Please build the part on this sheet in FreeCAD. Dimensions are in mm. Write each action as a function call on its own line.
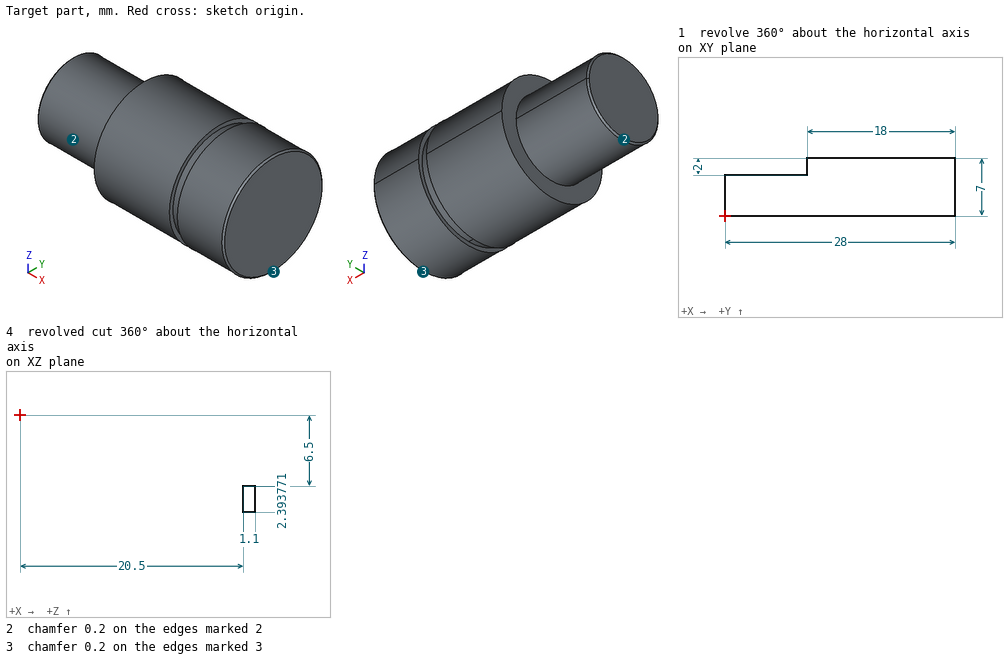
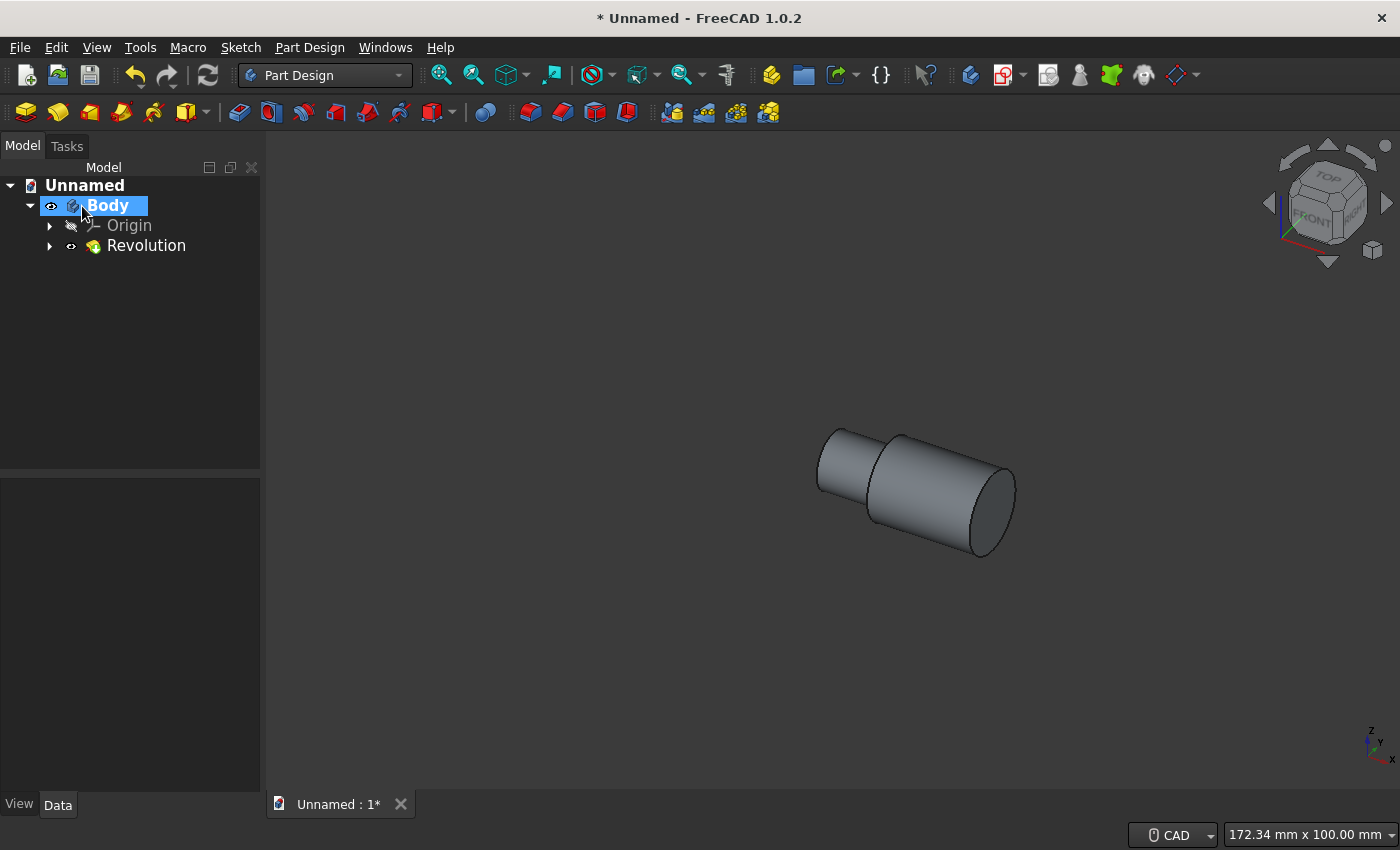
key(v)
key(f)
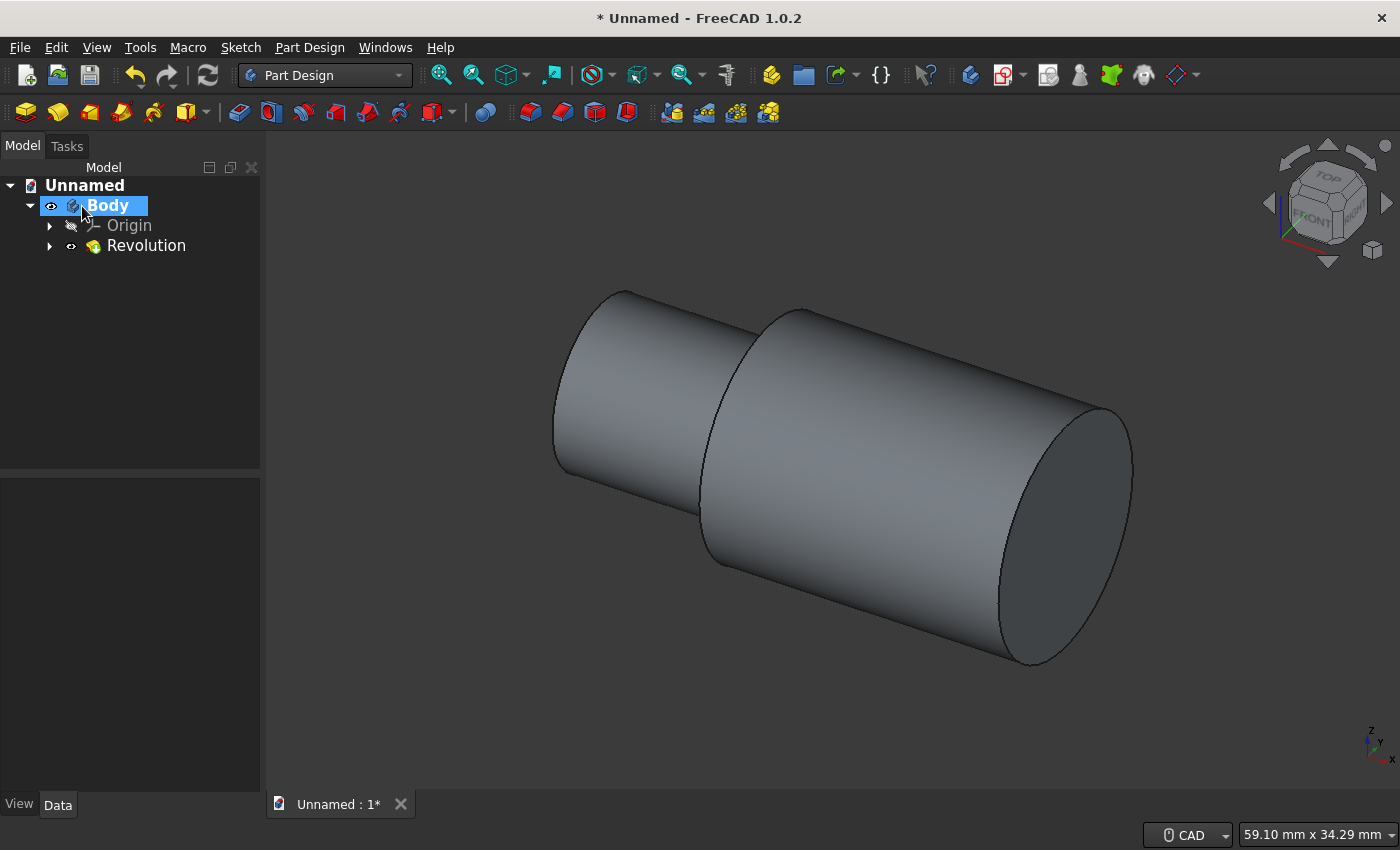
key(0)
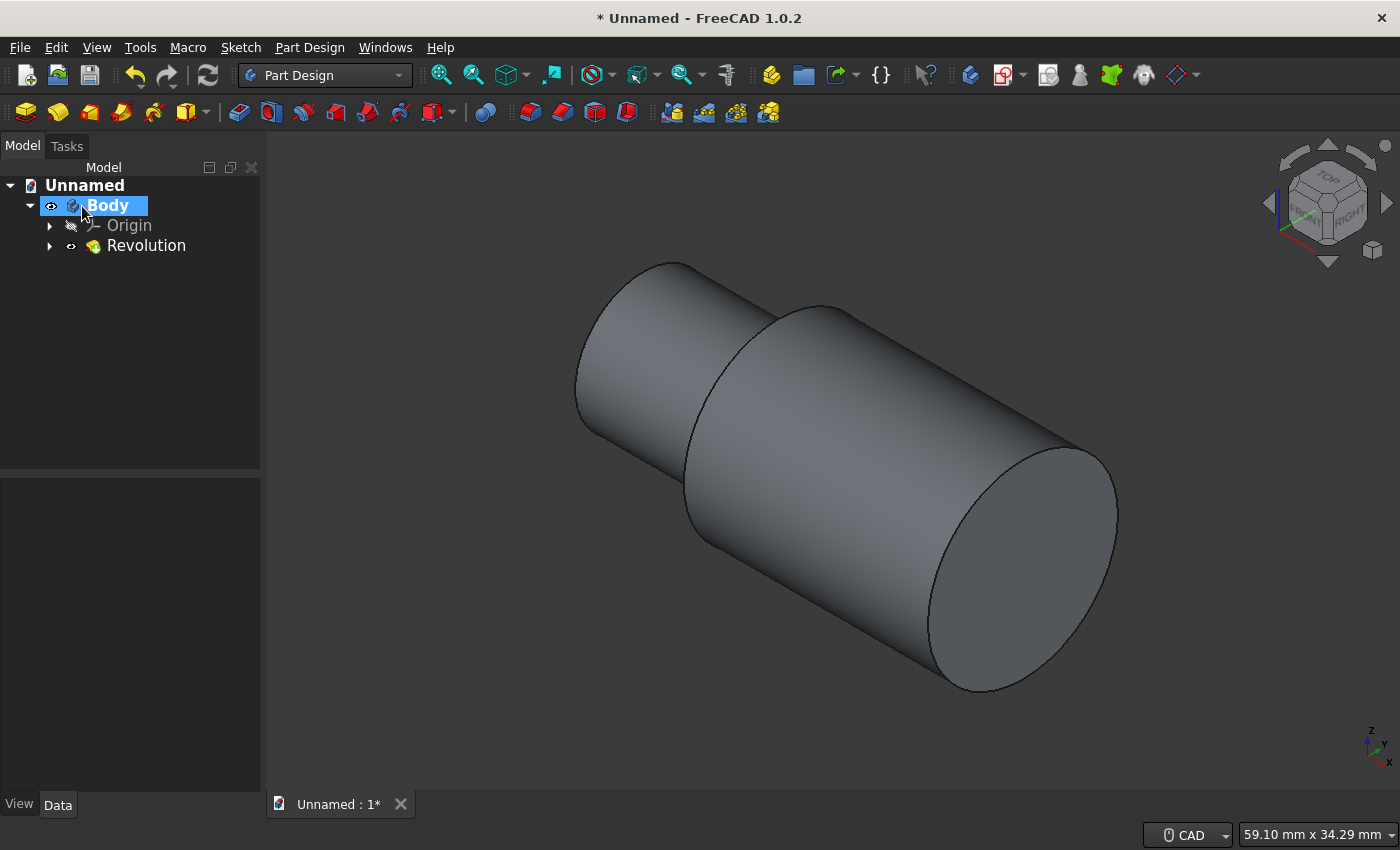
key(2)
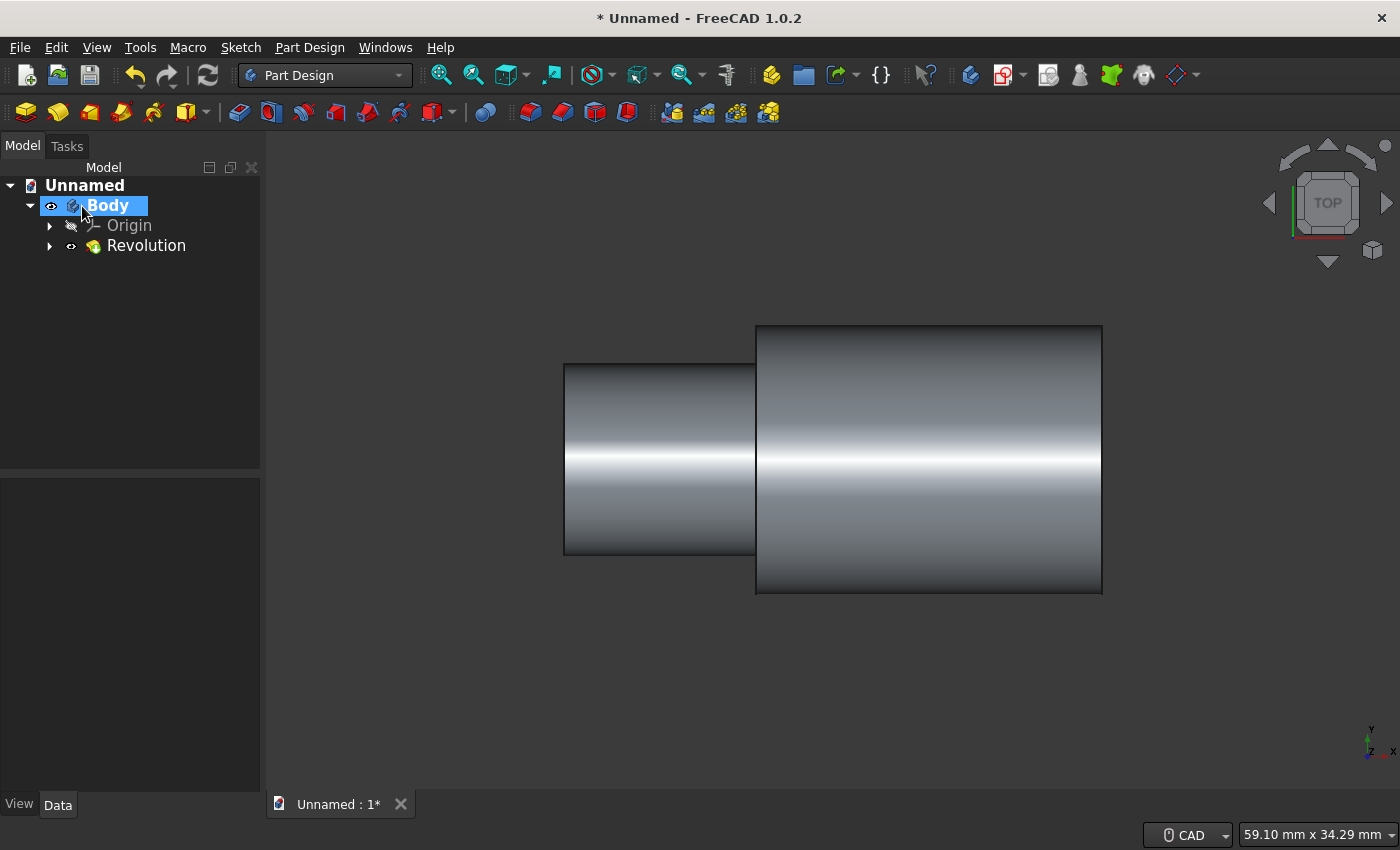
click(564, 537)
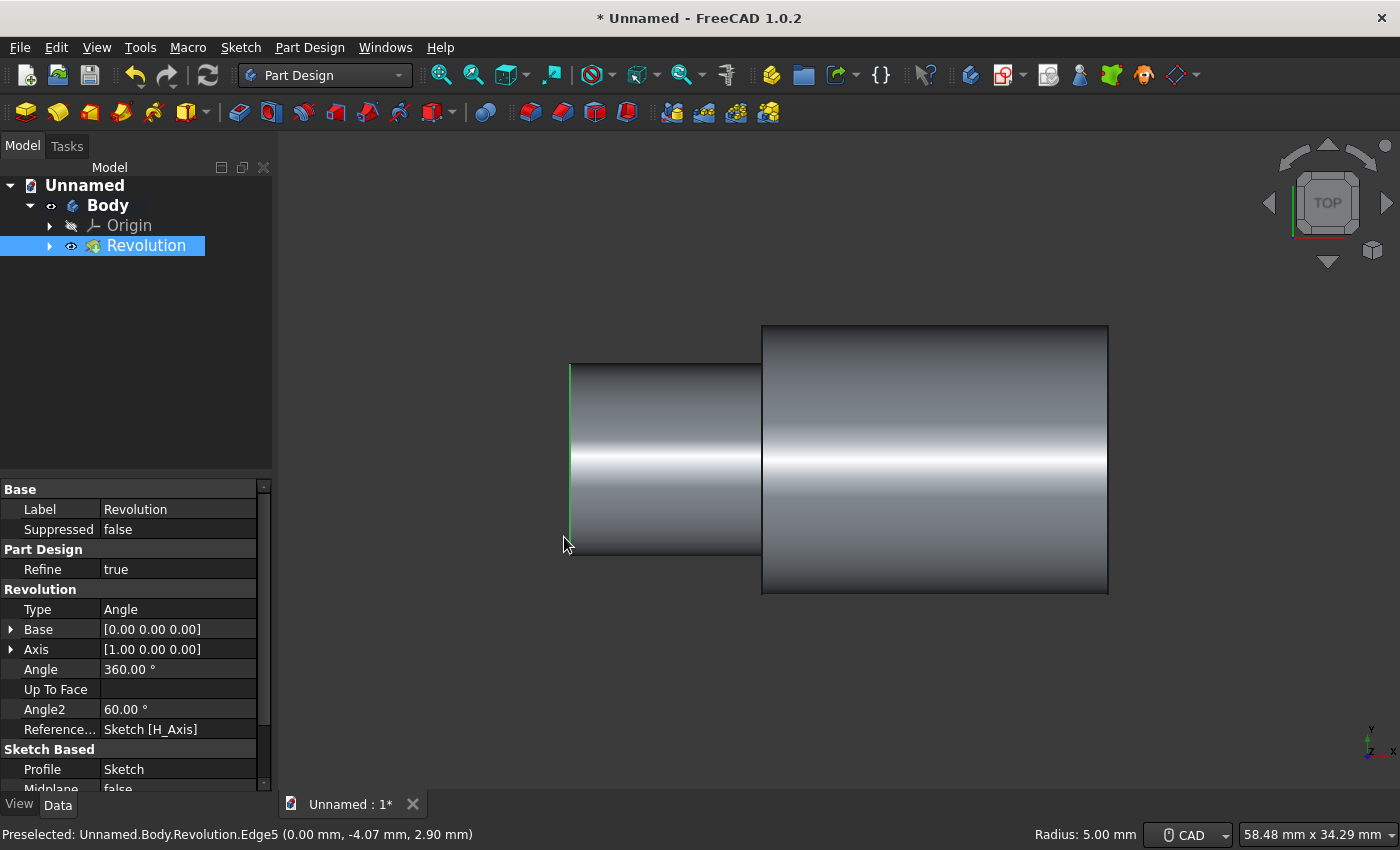
click(564, 112)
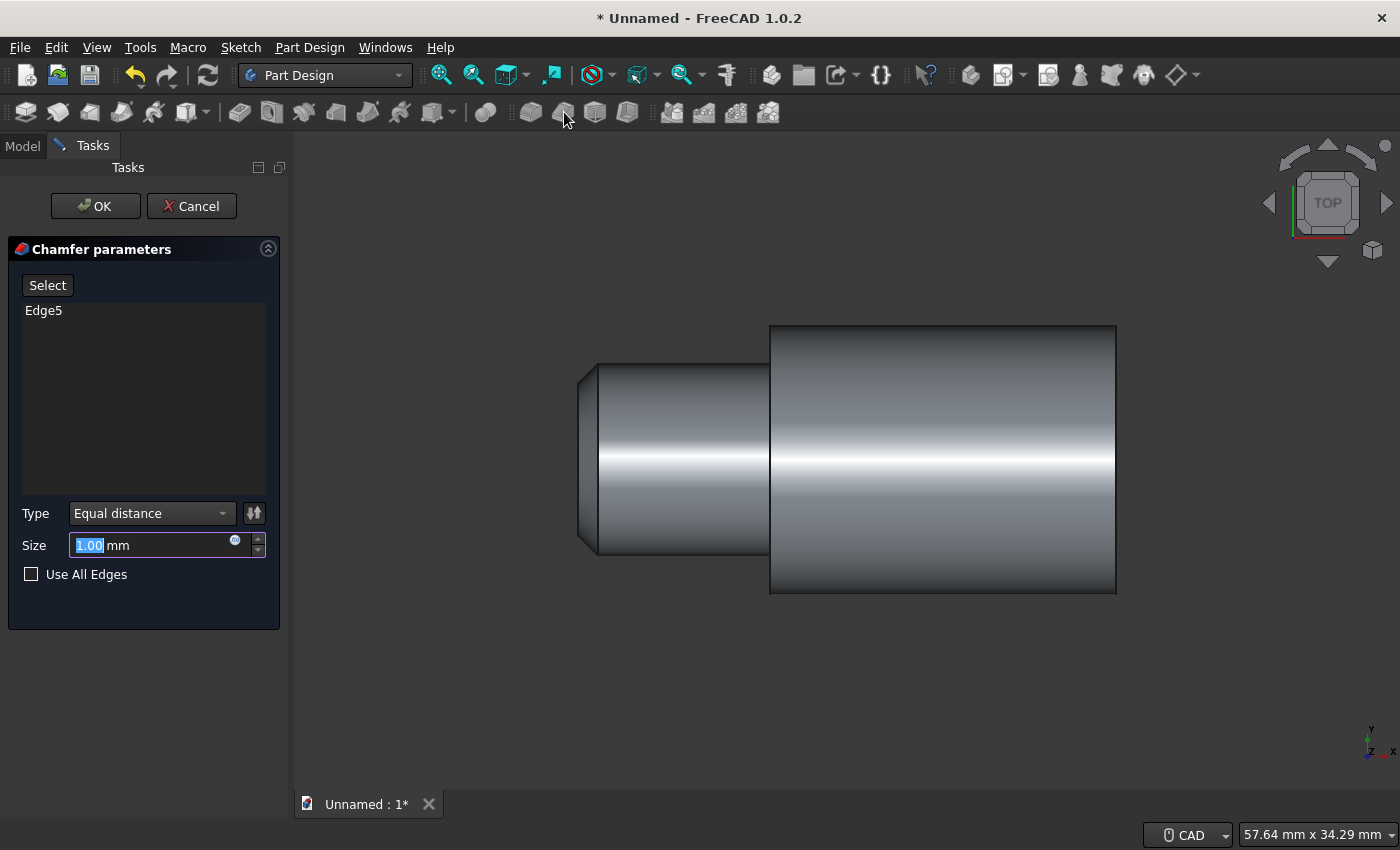
text(0.2)
key(Tab)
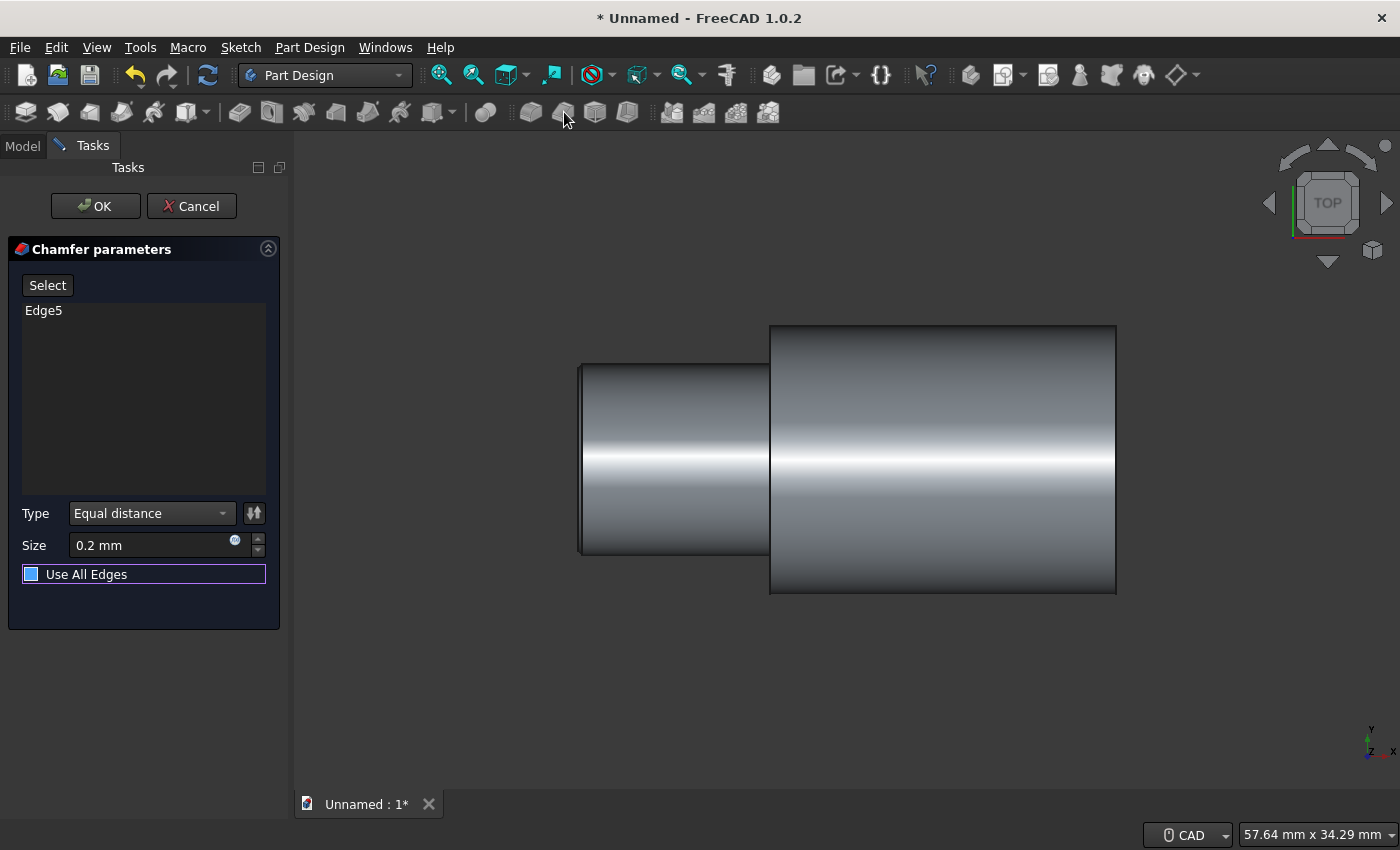
click(96, 206)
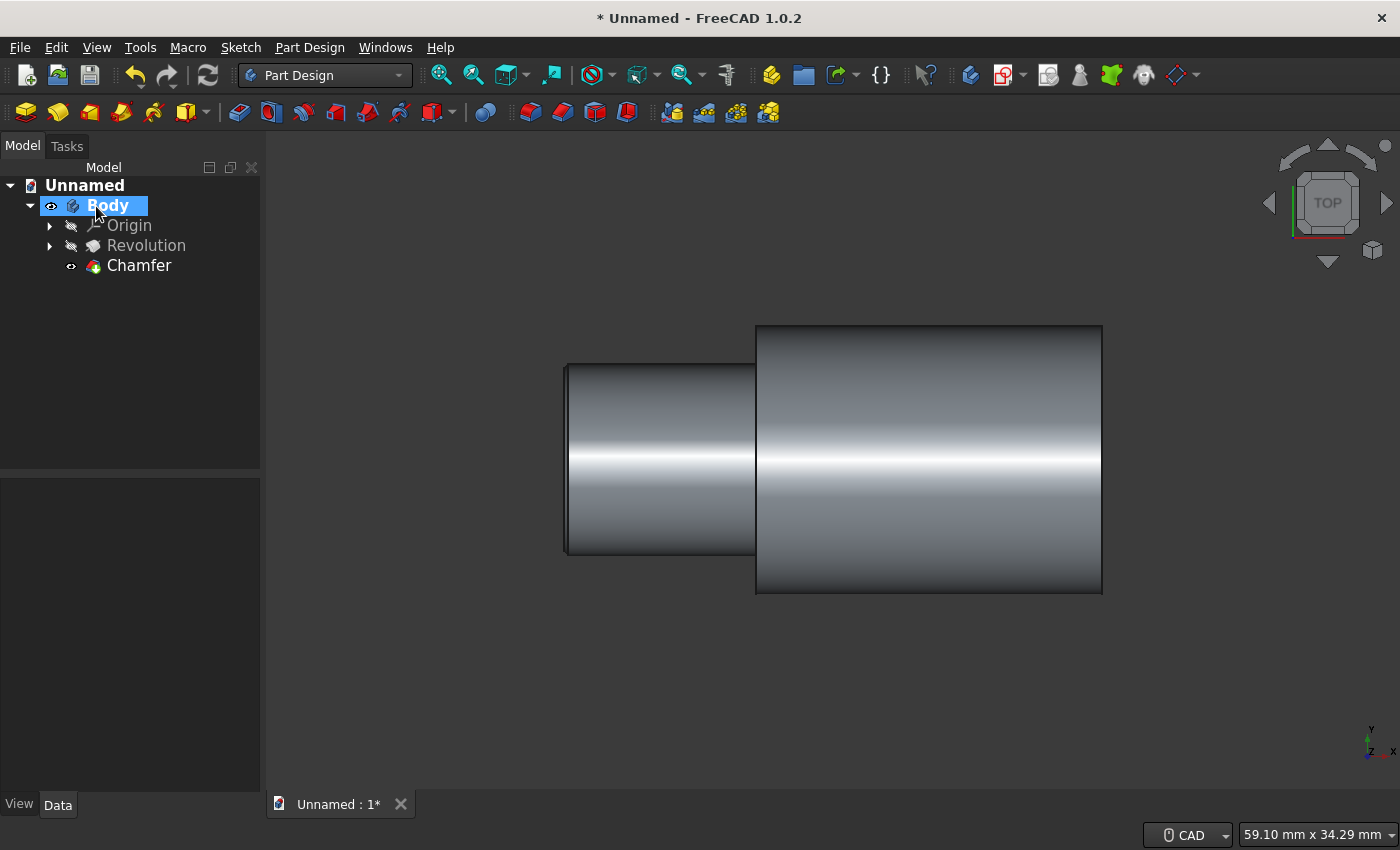
click(1102, 568)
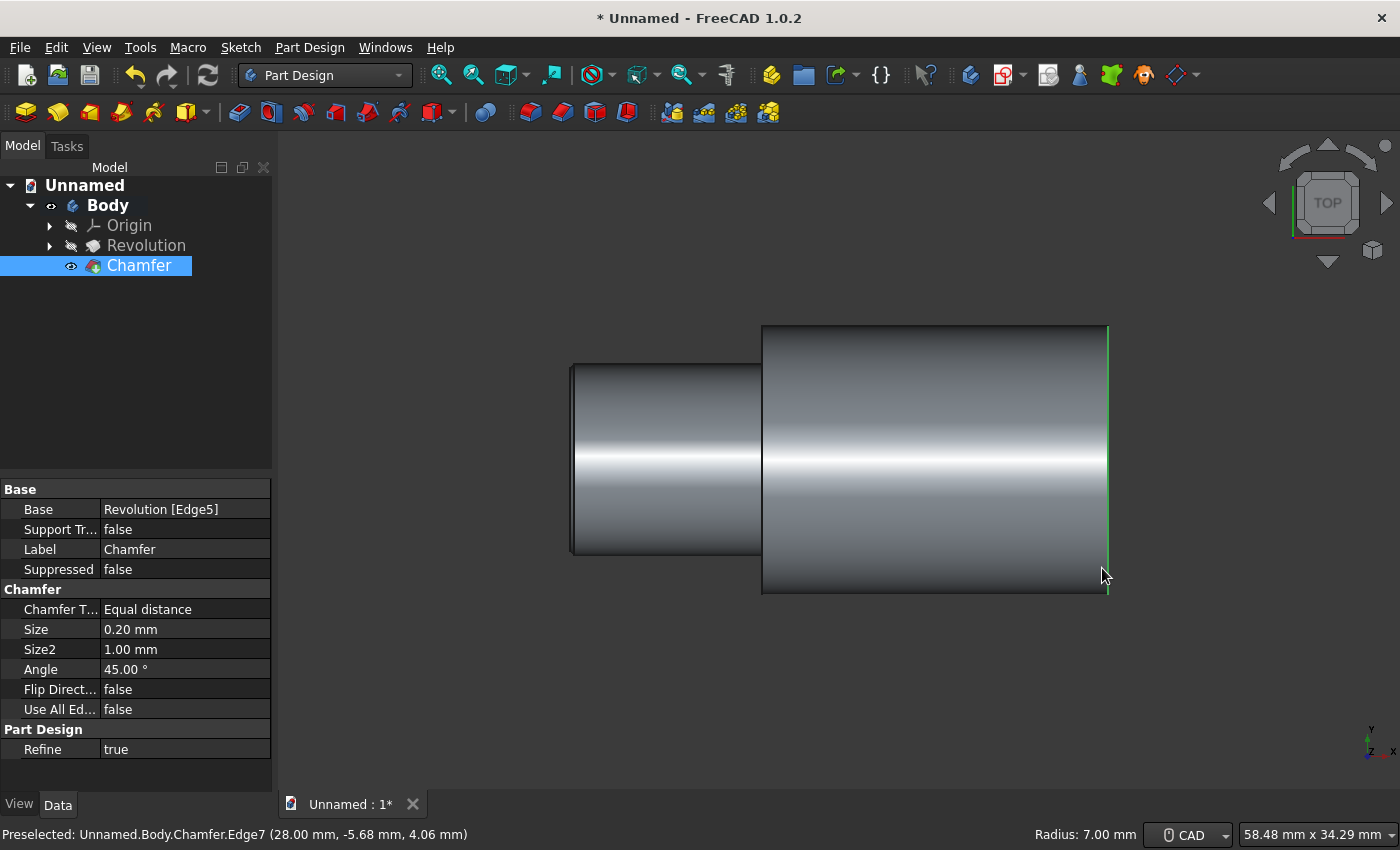
click(564, 112)